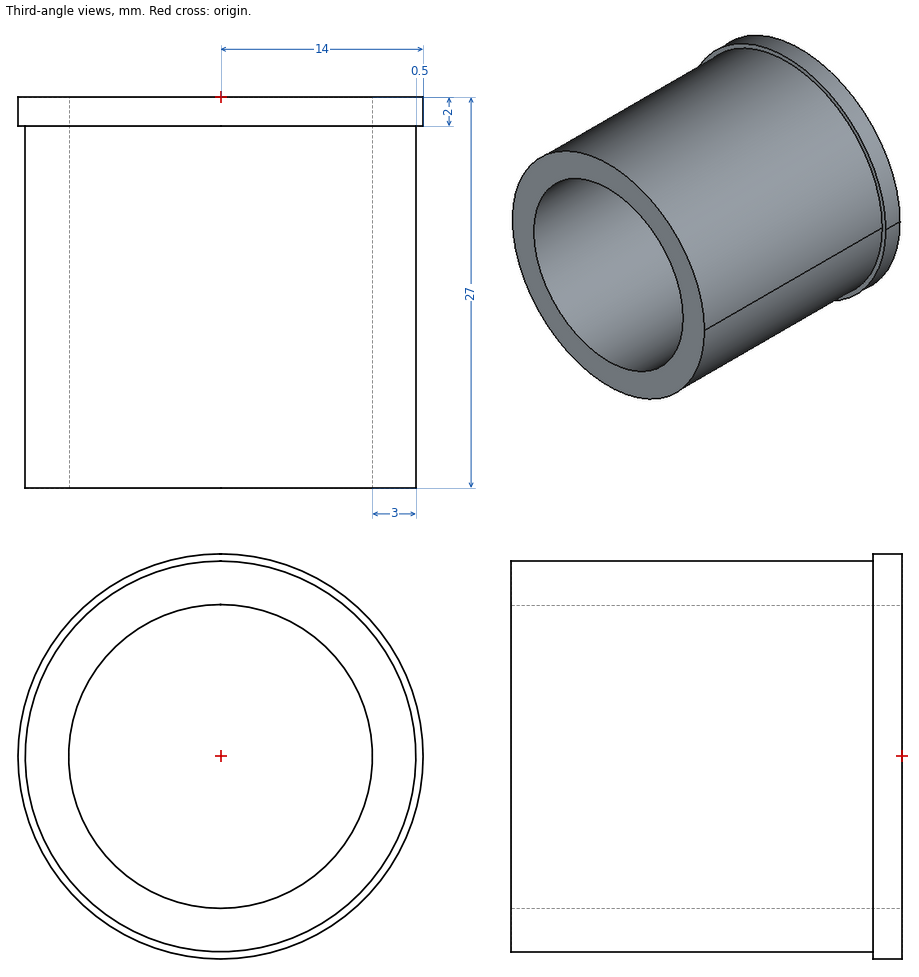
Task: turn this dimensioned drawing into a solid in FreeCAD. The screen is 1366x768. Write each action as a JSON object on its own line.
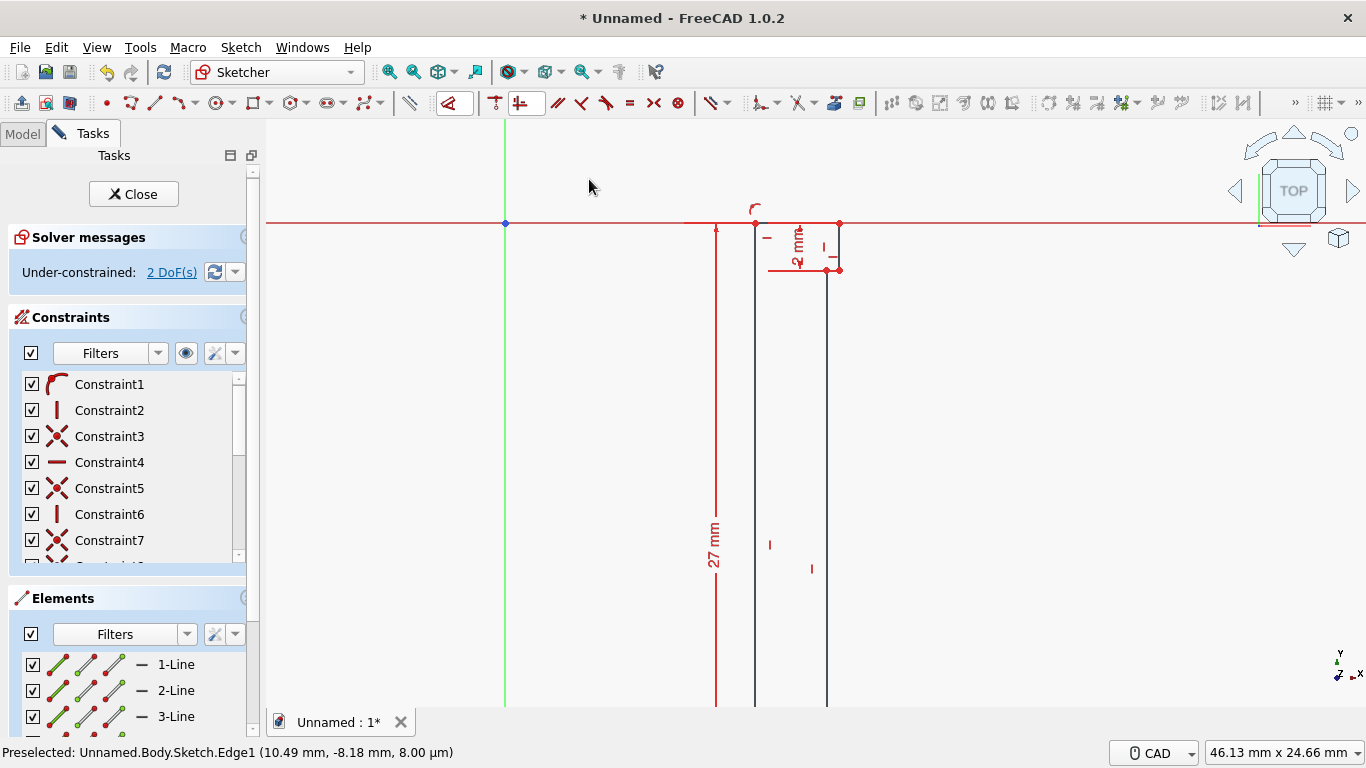
{"action": "scroll", "coordinate": [833, 271], "scroll_direction": "up", "scroll_amount": 7}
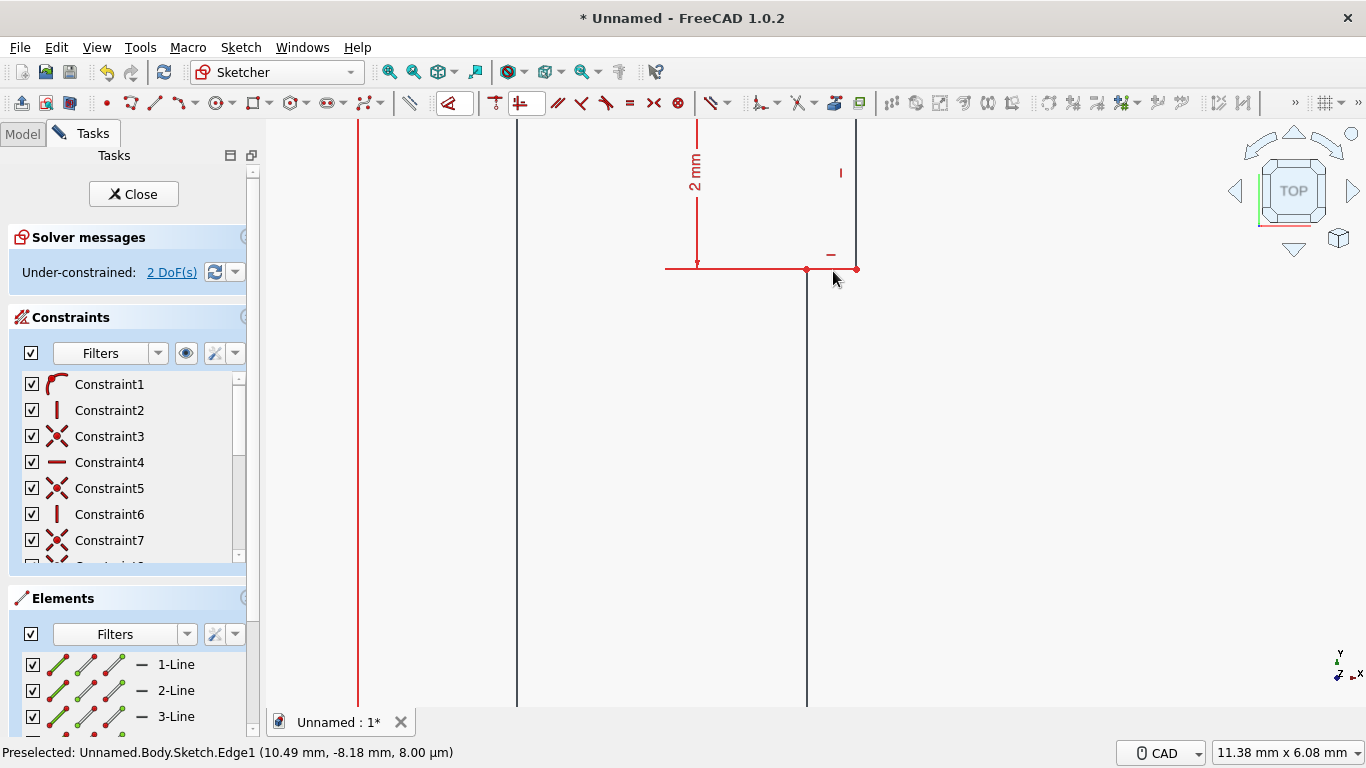
{"action": "left_click", "coordinate": [832, 269]}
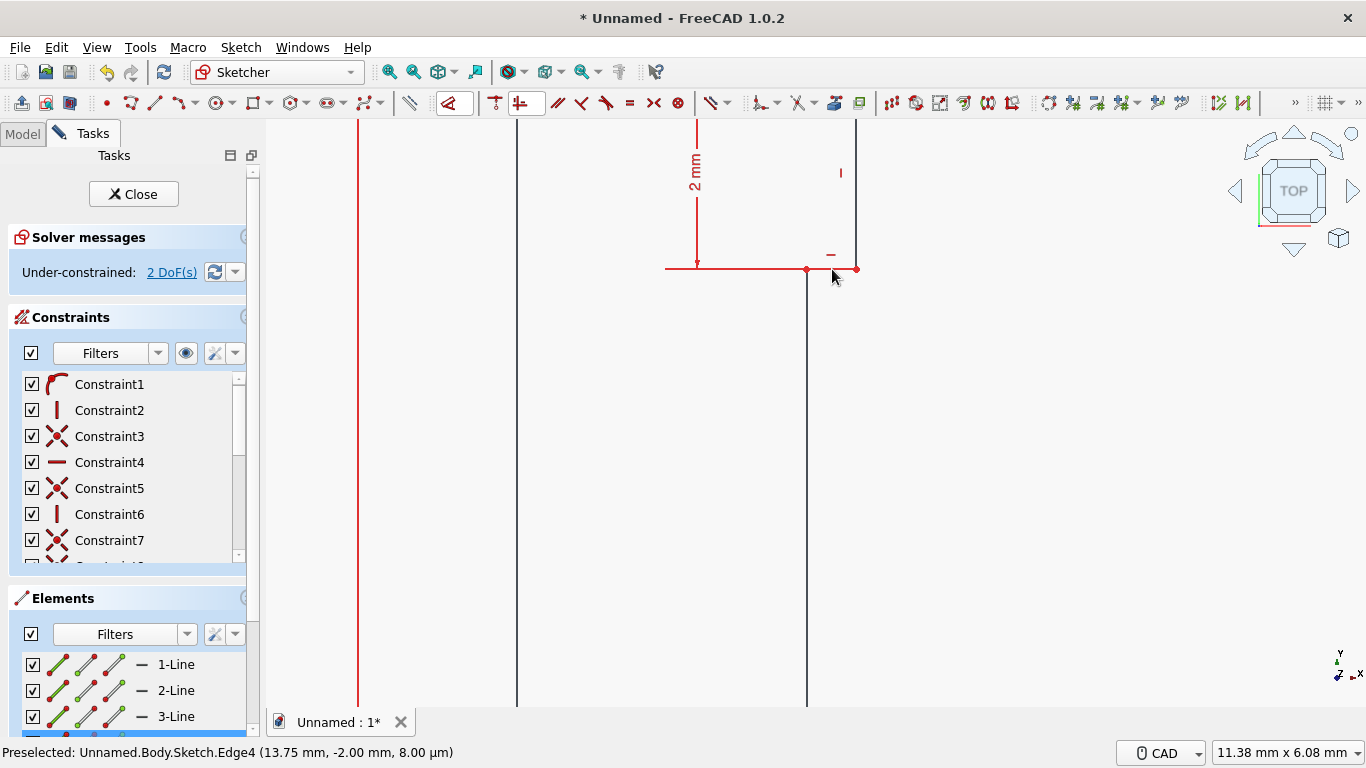
{"action": "key", "text": "l"}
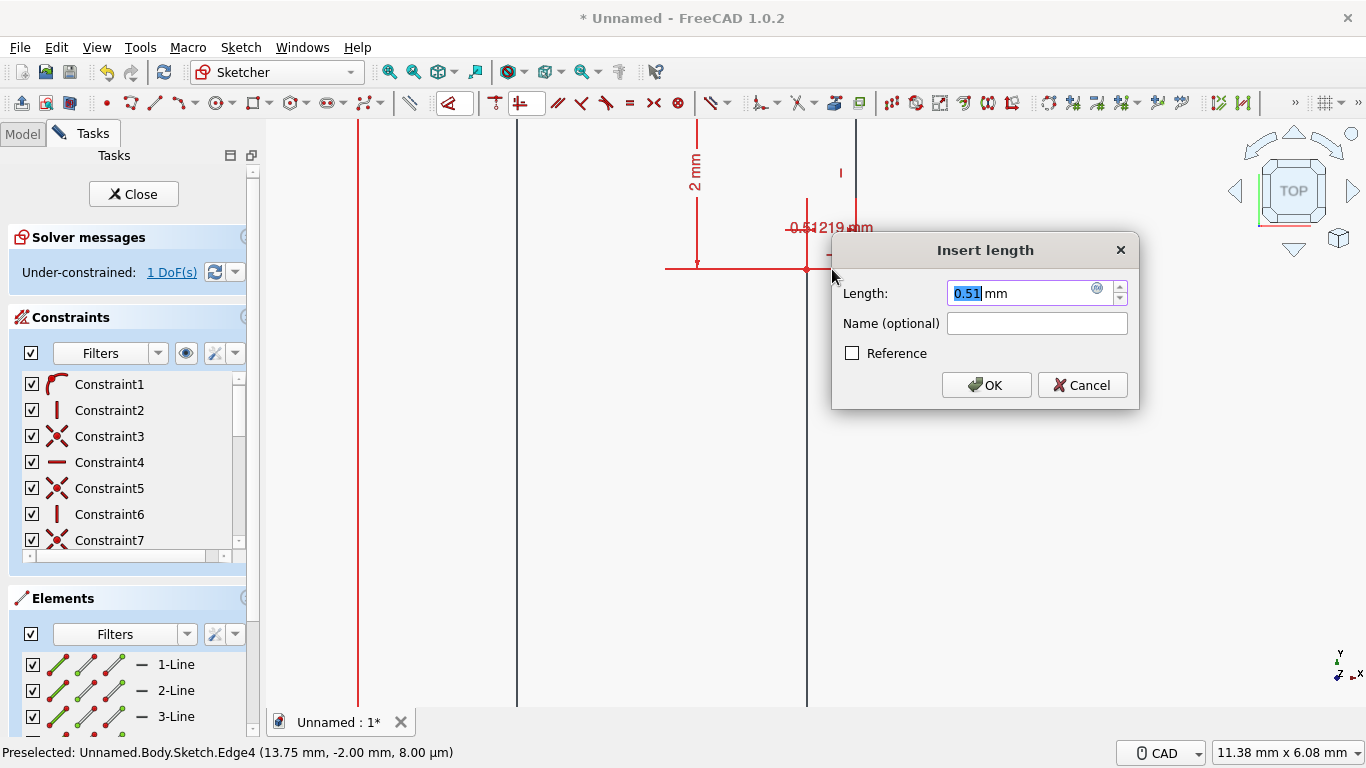
{"action": "type", "text": "0.5"}
{"action": "key", "text": "Return"}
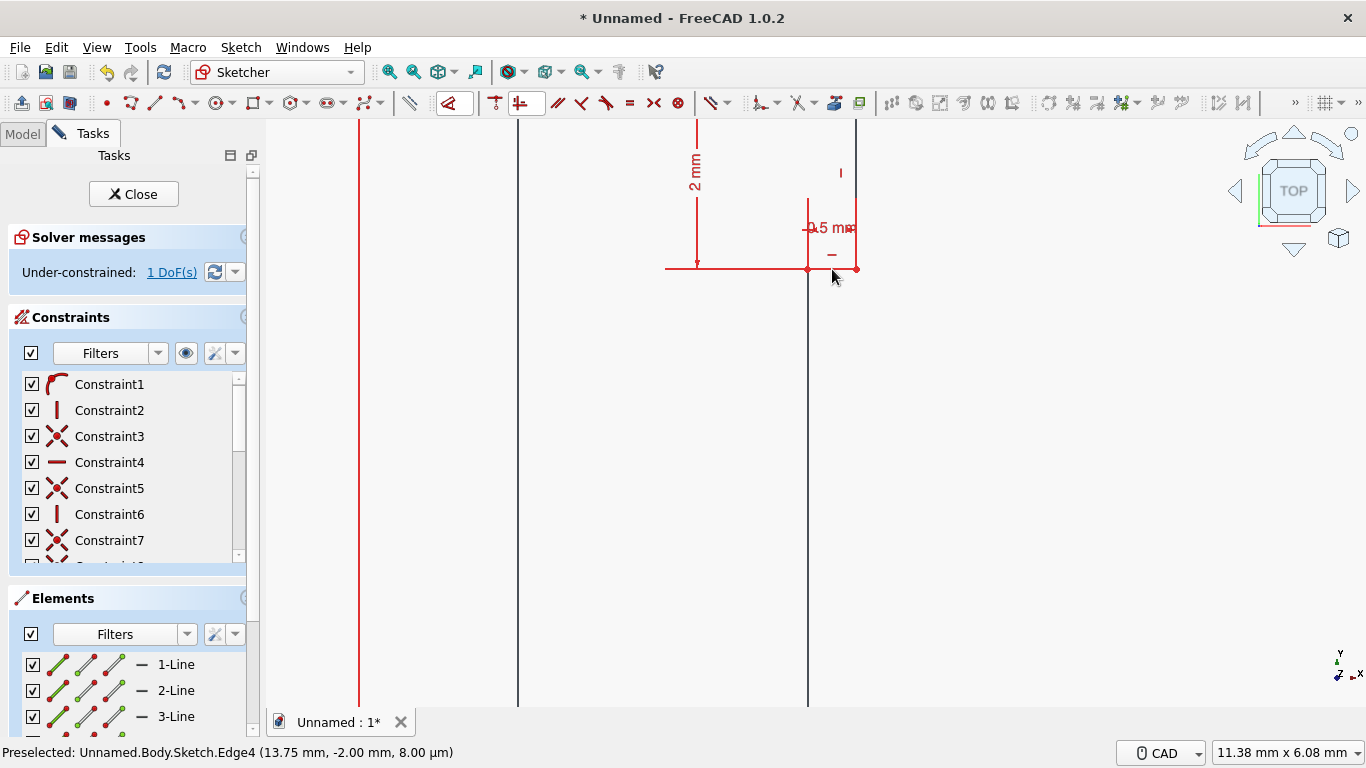
{"action": "scroll", "coordinate": [836, 261], "scroll_direction": "down", "scroll_amount": 10}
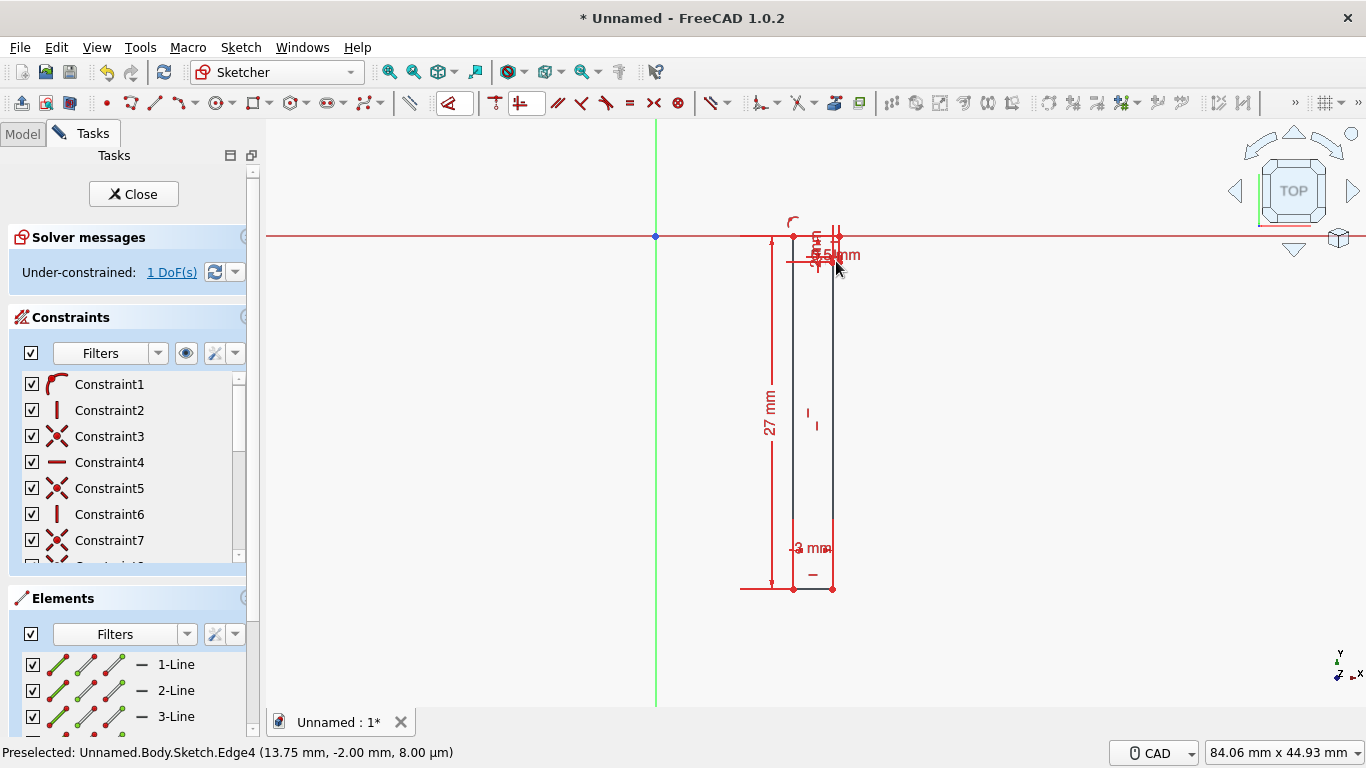
{"action": "scroll", "coordinate": [839, 262], "scroll_direction": "up", "scroll_amount": 4}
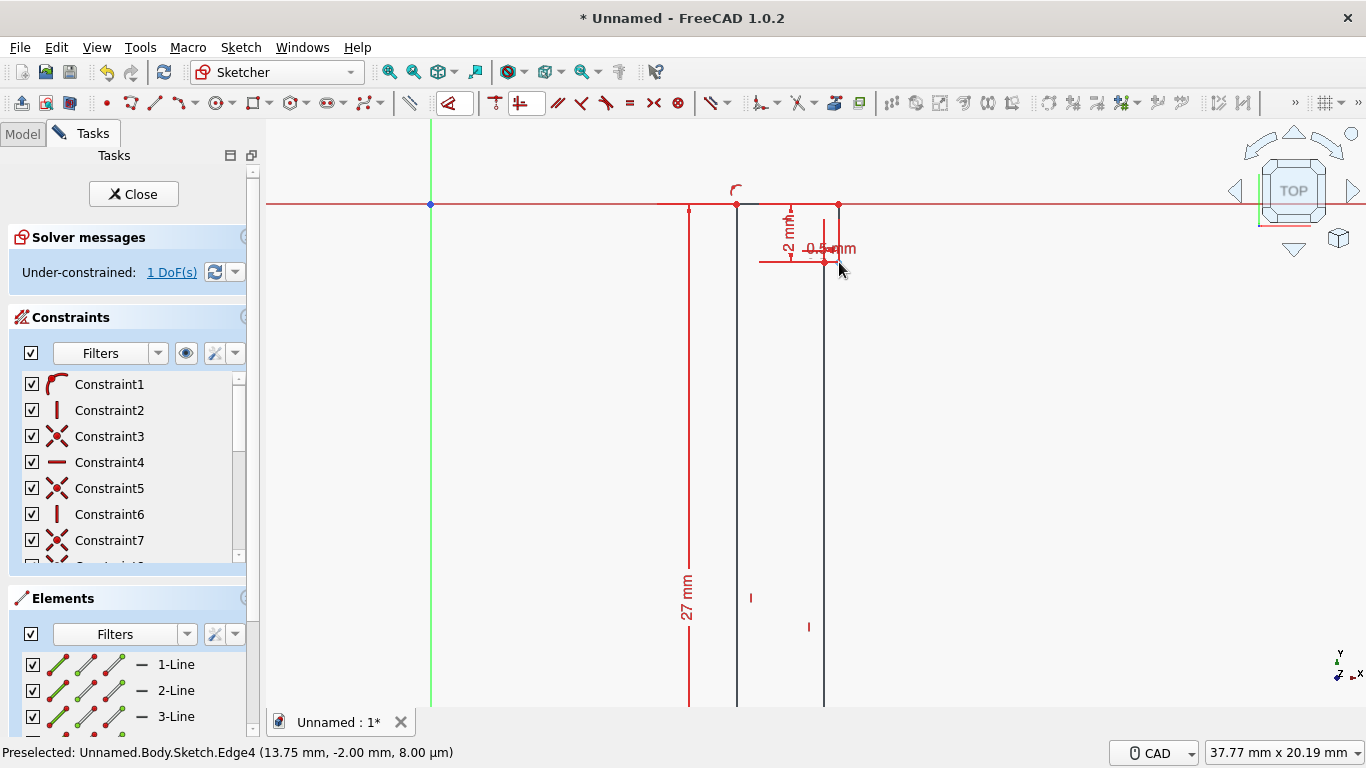
{"action": "left_click", "coordinate": [839, 262]}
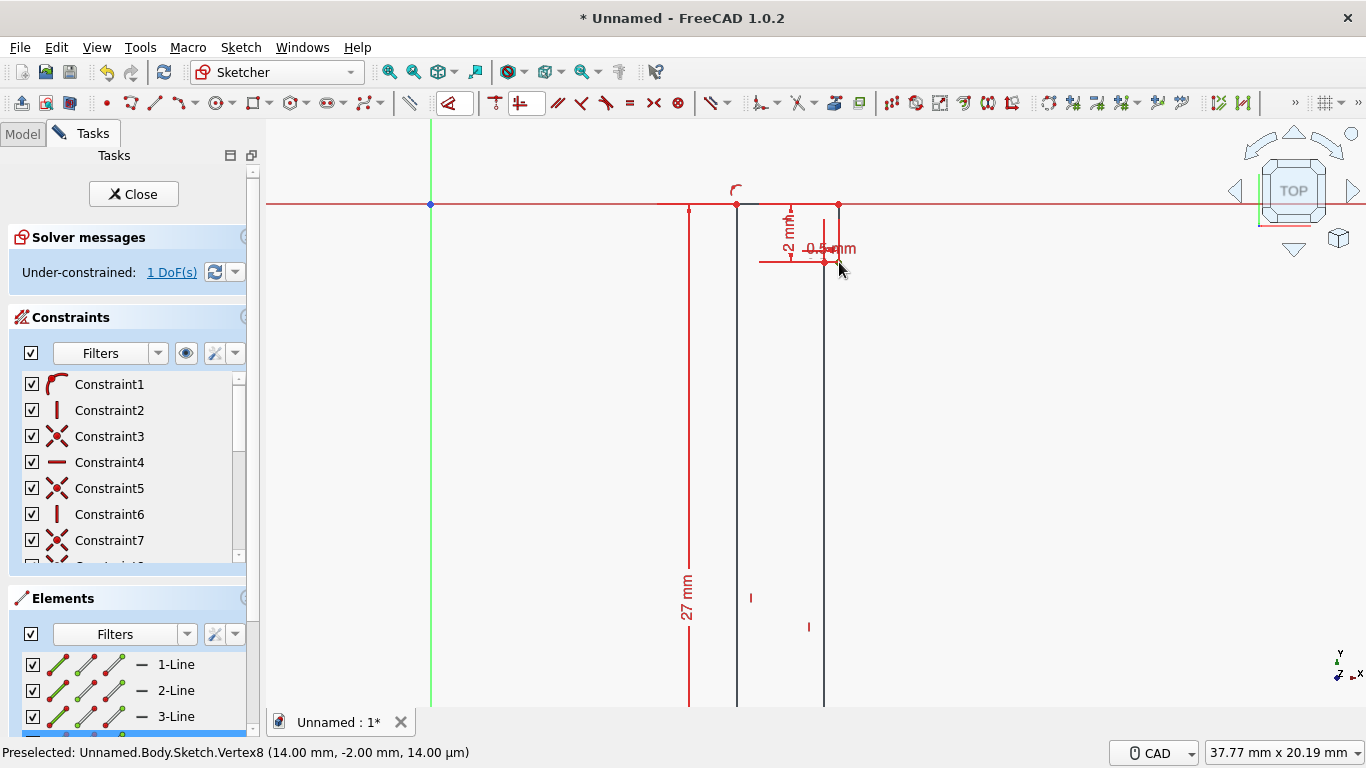
{"action": "key", "text": "l"}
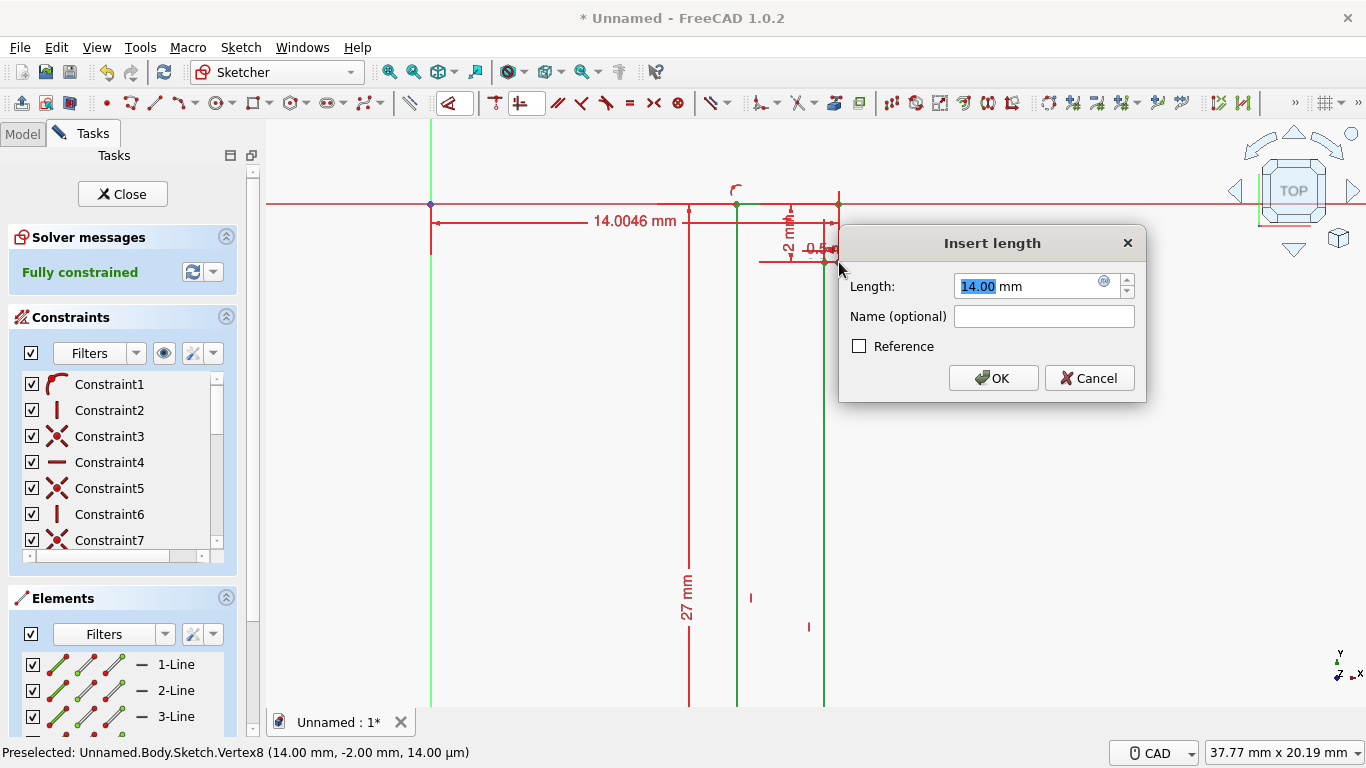
{"action": "type", "text": "14"}
{"action": "key", "text": "Return"}